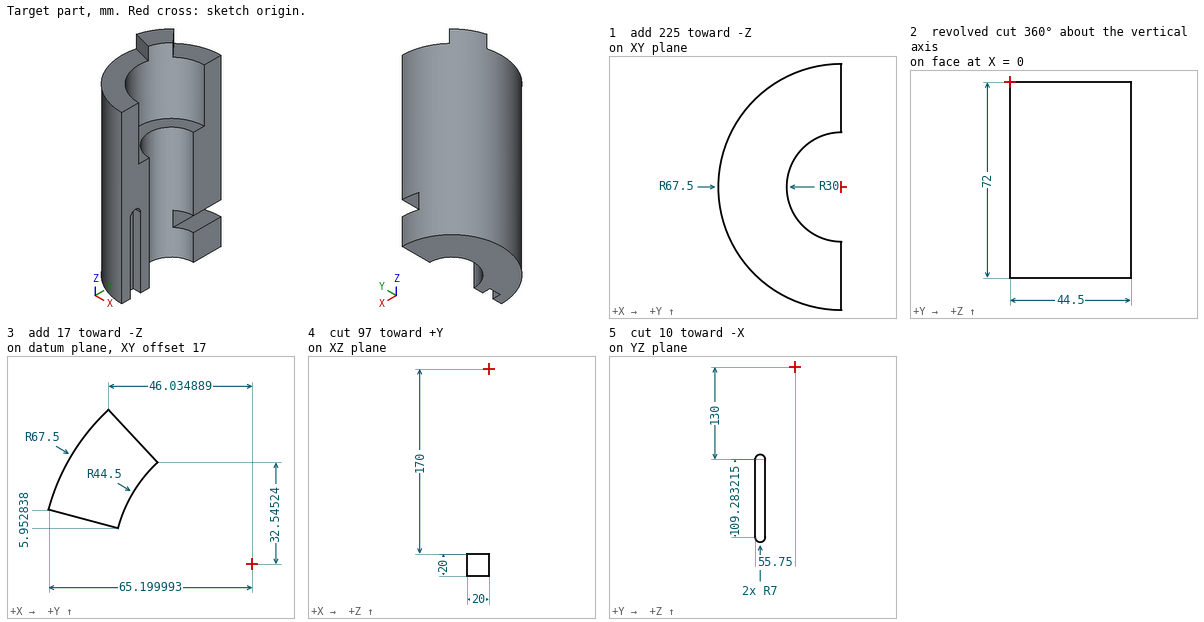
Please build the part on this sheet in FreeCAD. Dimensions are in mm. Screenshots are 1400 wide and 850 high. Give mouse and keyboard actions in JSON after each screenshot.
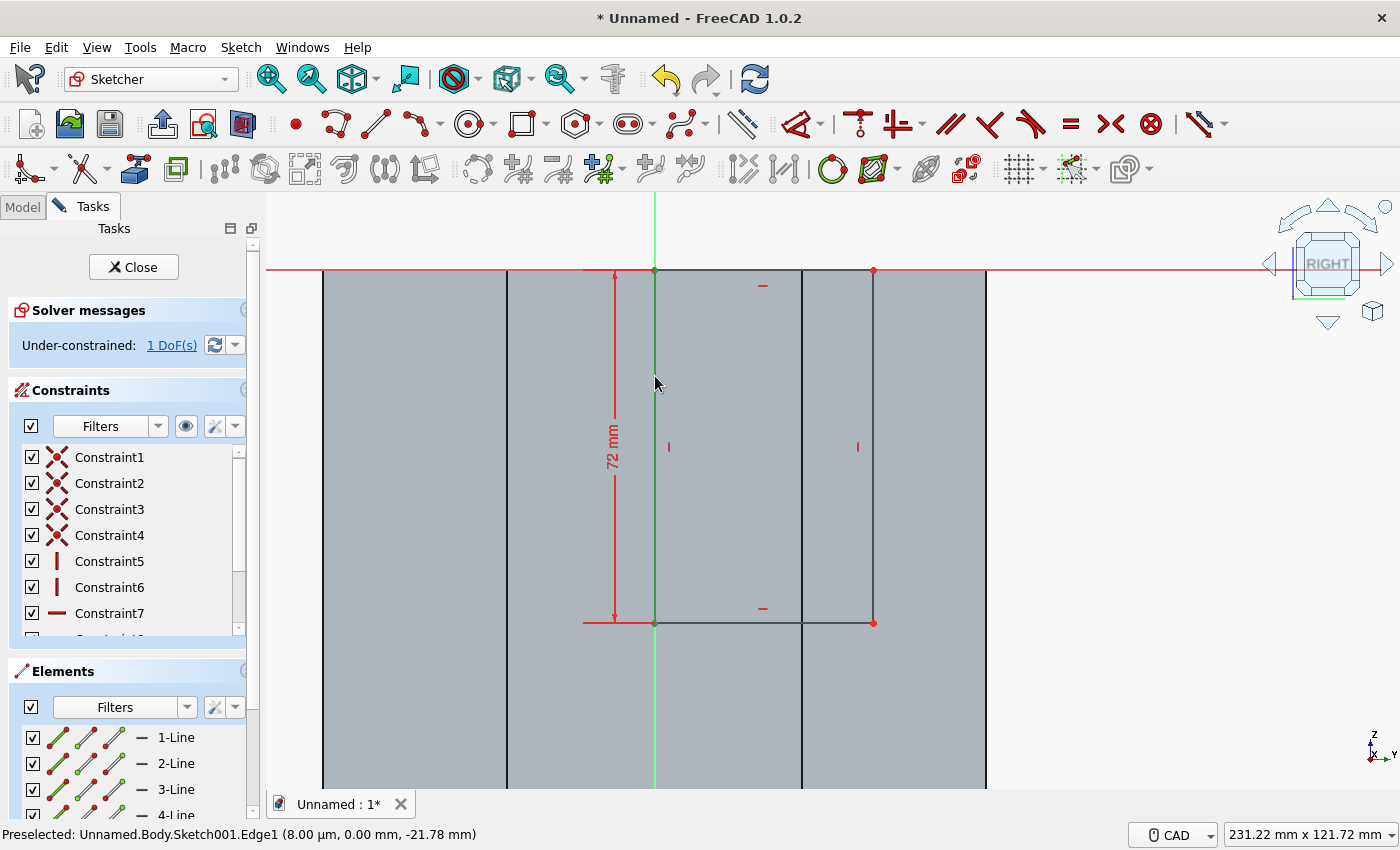
{"action": "left_click", "coordinate": [720, 623]}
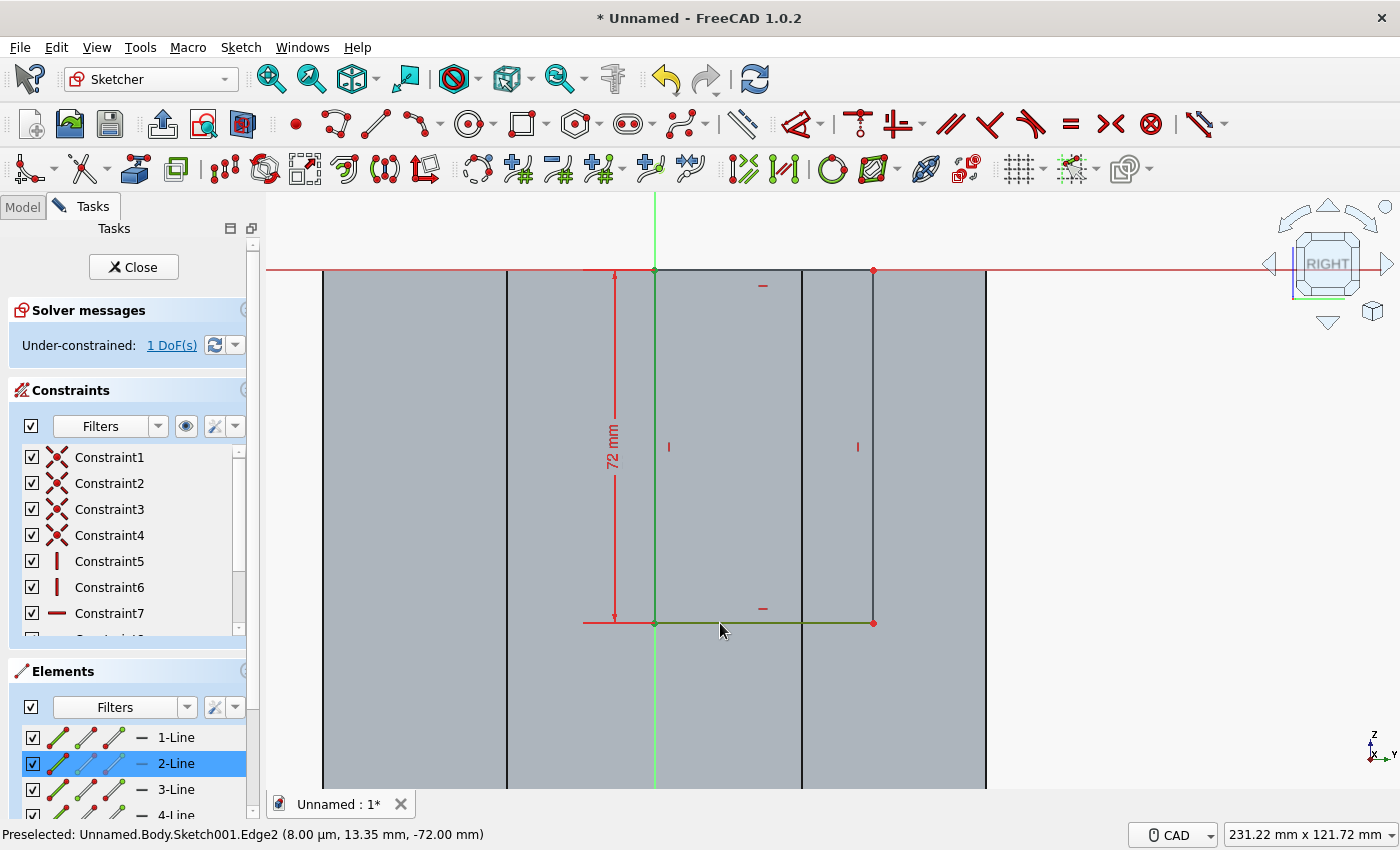
{"action": "key", "text": "l"}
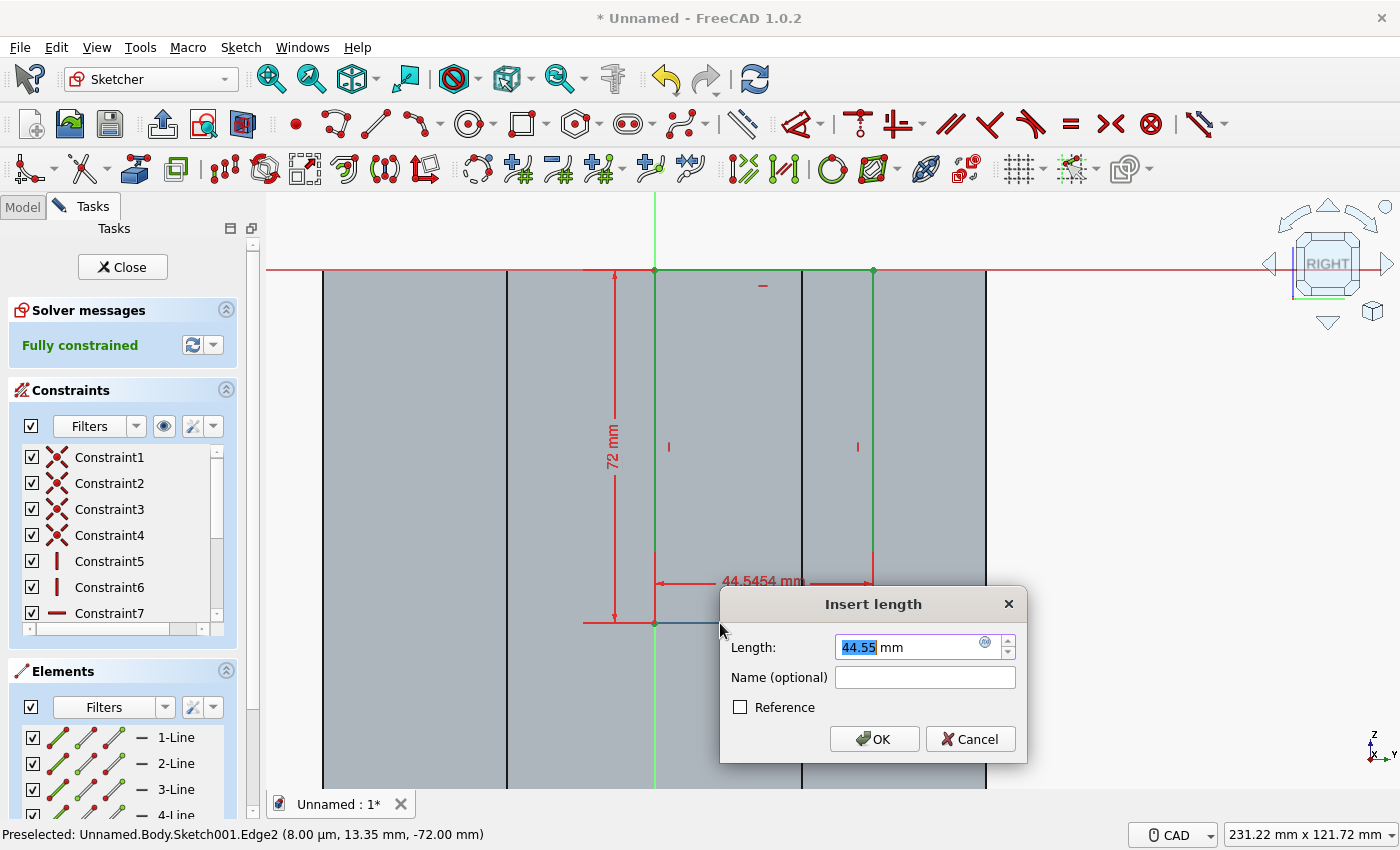
{"action": "type", "text": "44.5"}
{"action": "key", "text": "Return"}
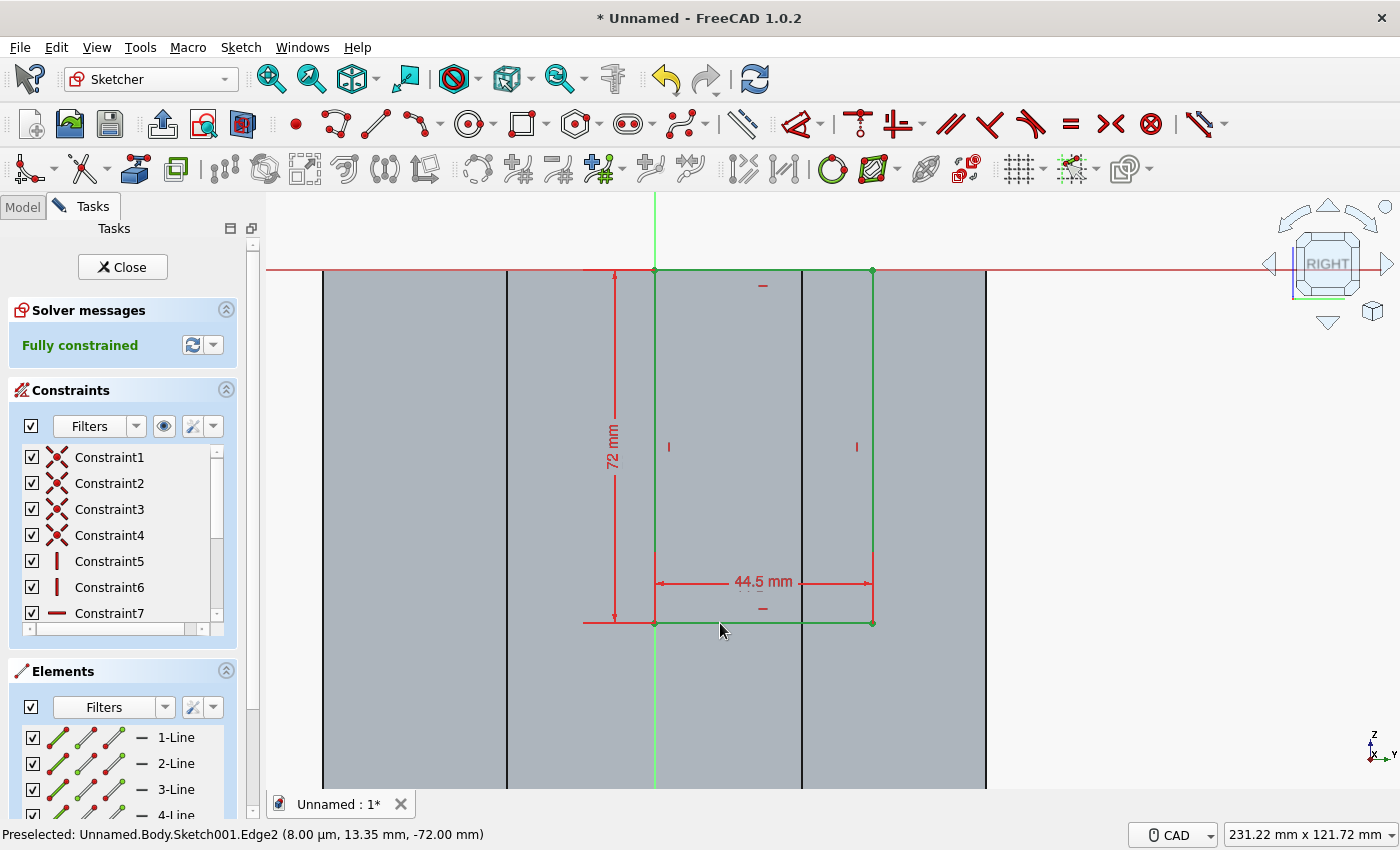
{"action": "left_click", "coordinate": [123, 267]}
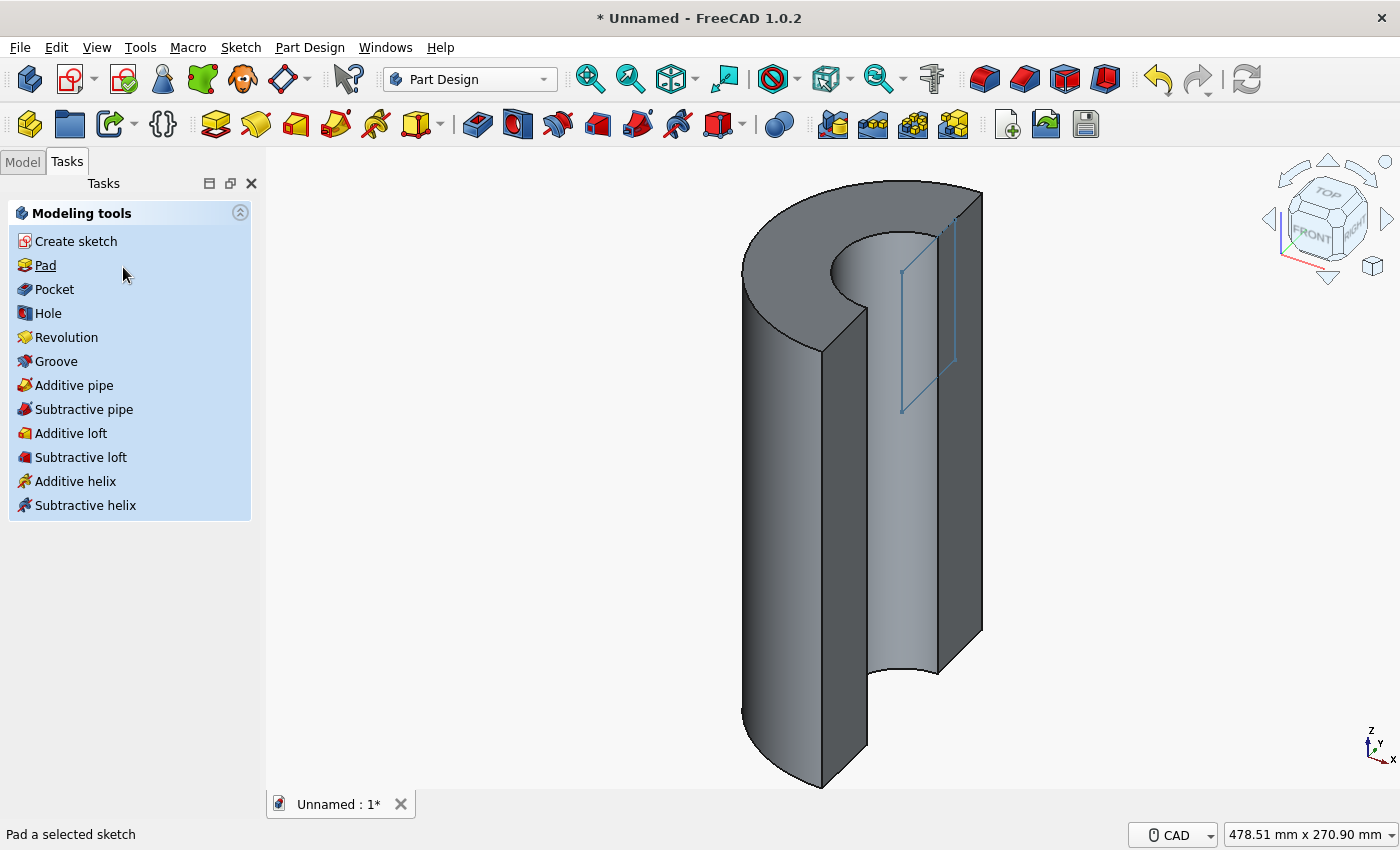
{"action": "left_click", "coordinate": [558, 124]}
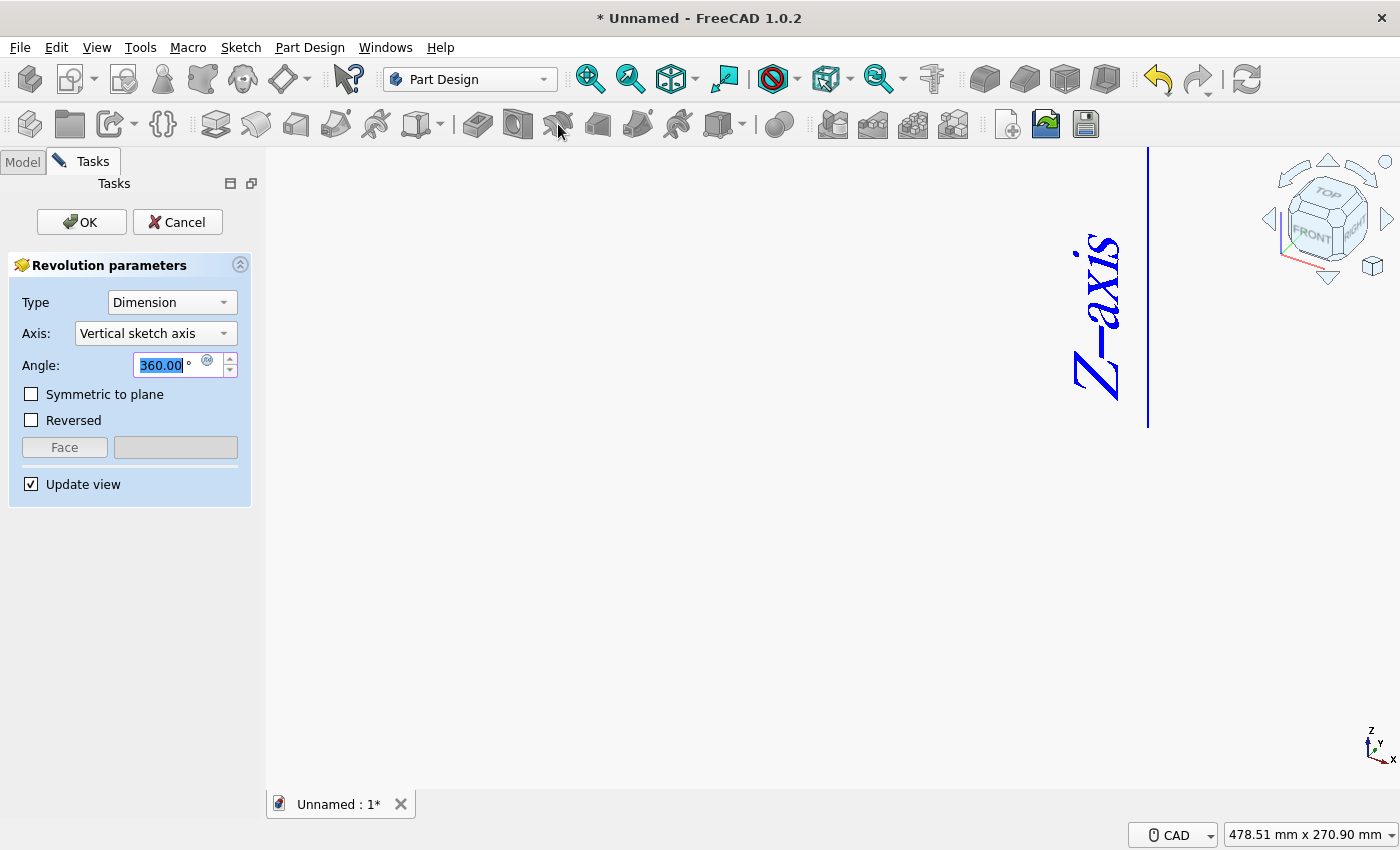
{"action": "left_click", "coordinate": [82, 222]}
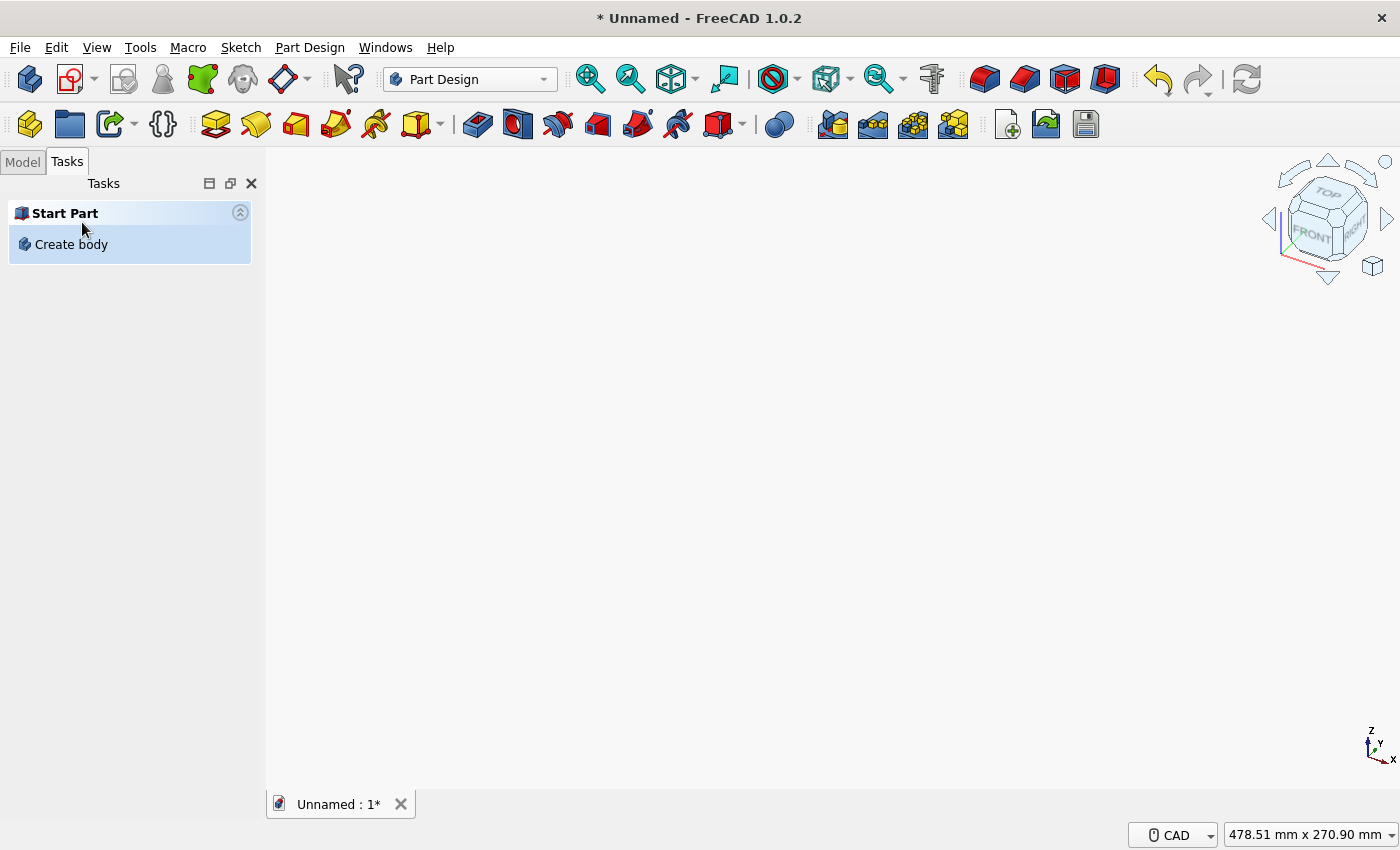
{"action": "key", "text": "v f"}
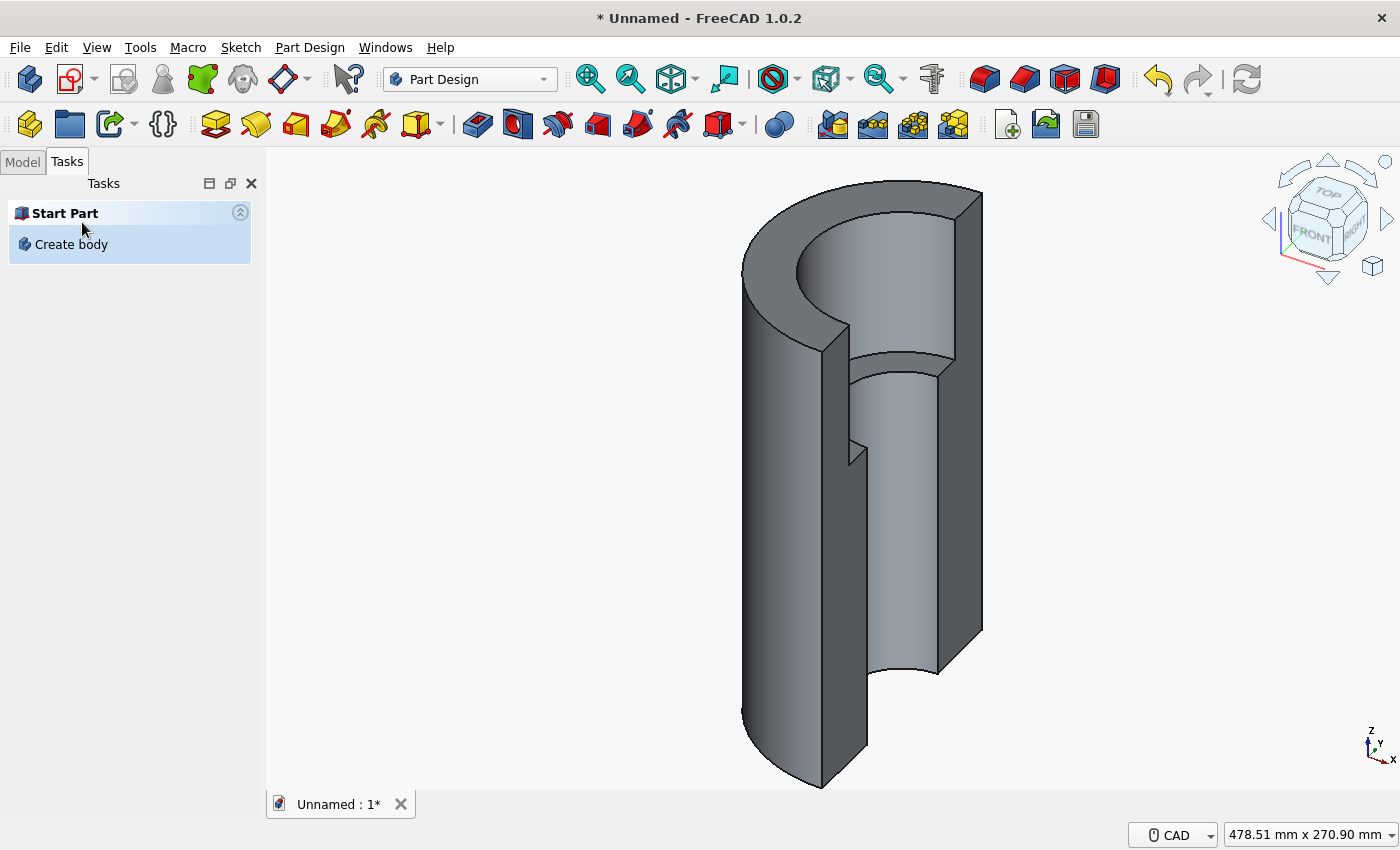
{"action": "left_click", "coordinate": [23, 161]}